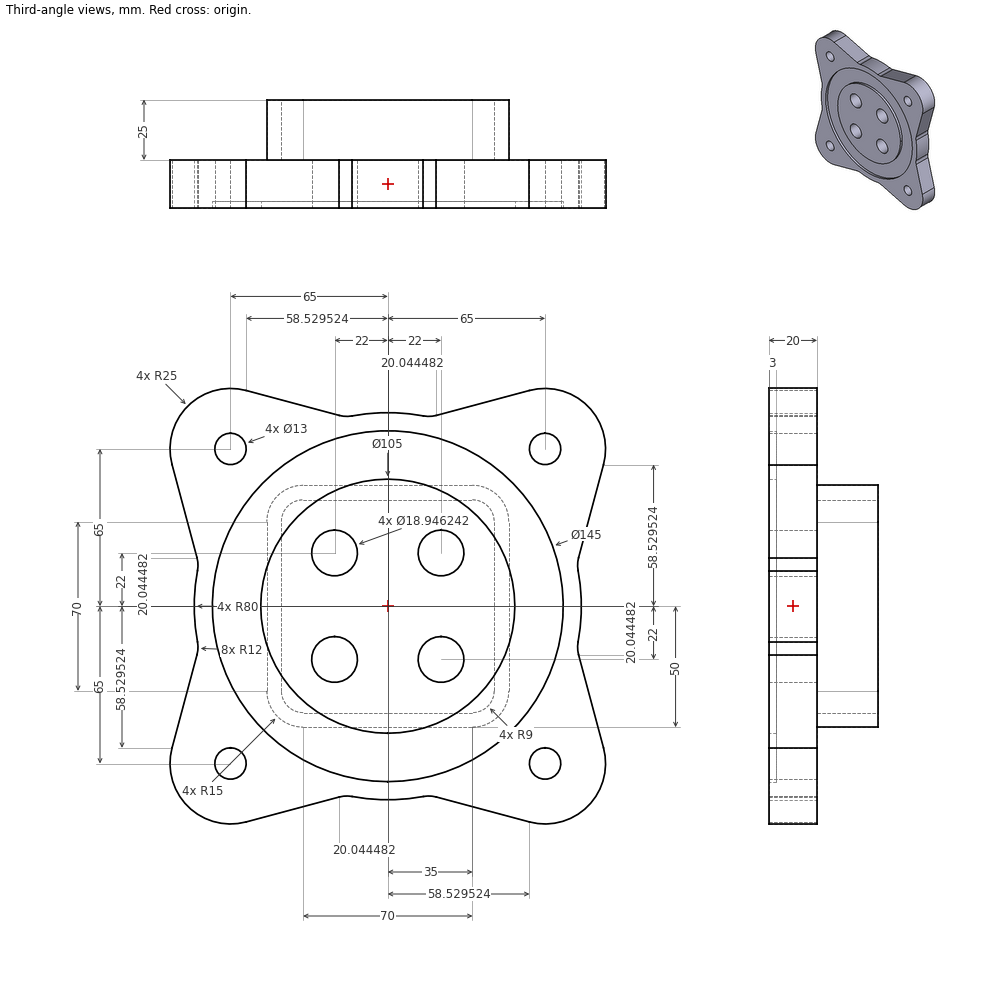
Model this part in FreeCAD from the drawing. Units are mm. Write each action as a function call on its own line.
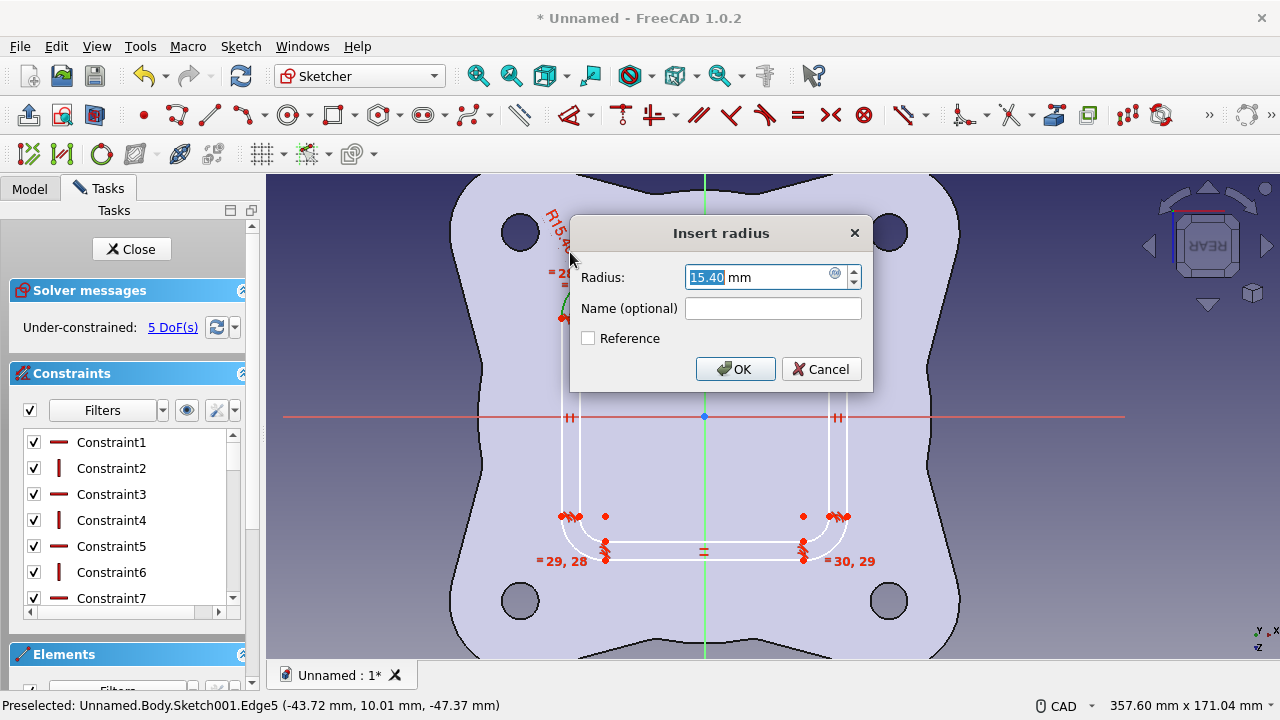
text(15)
key(Return)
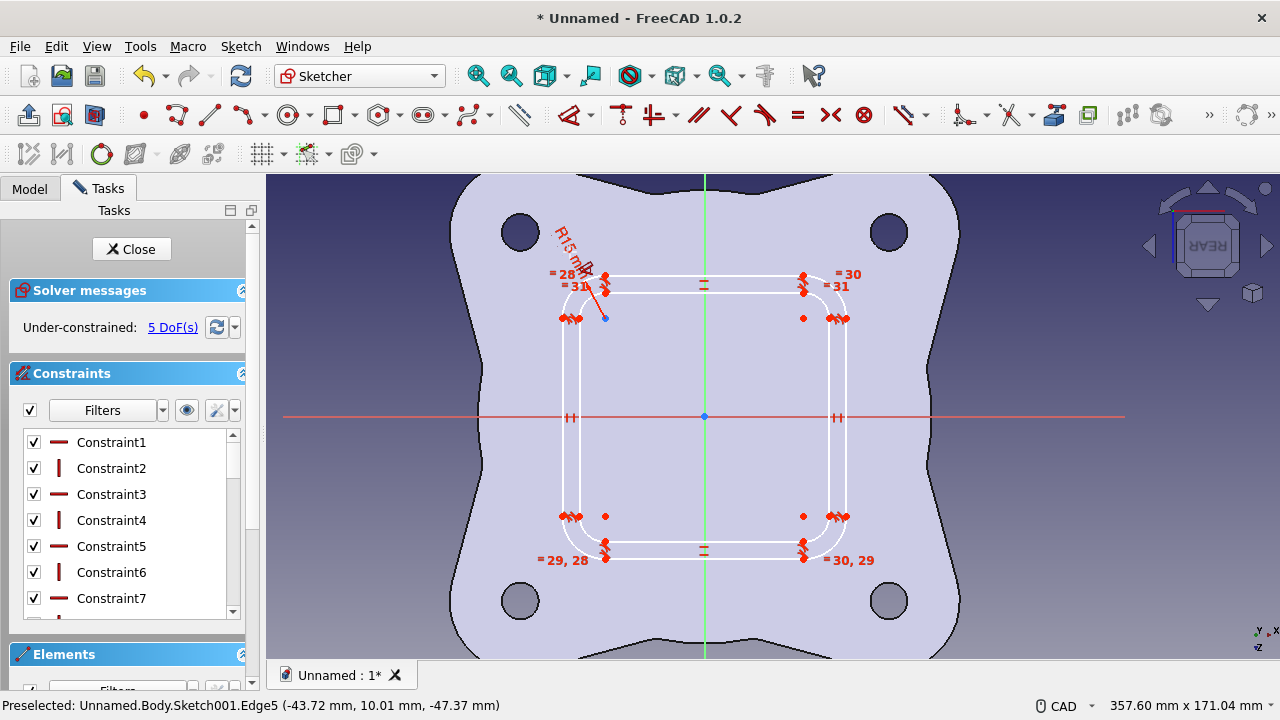
scroll(826, 307, up, 3)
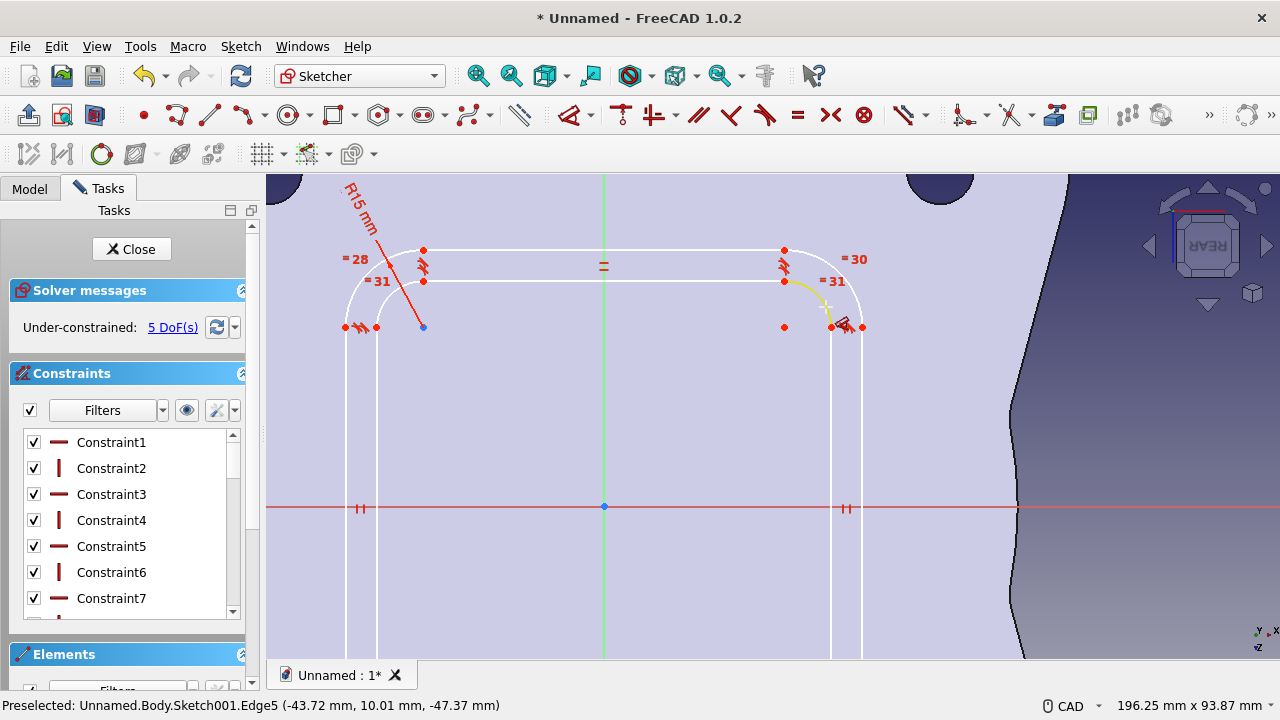
click(826, 307)
click(715, 363)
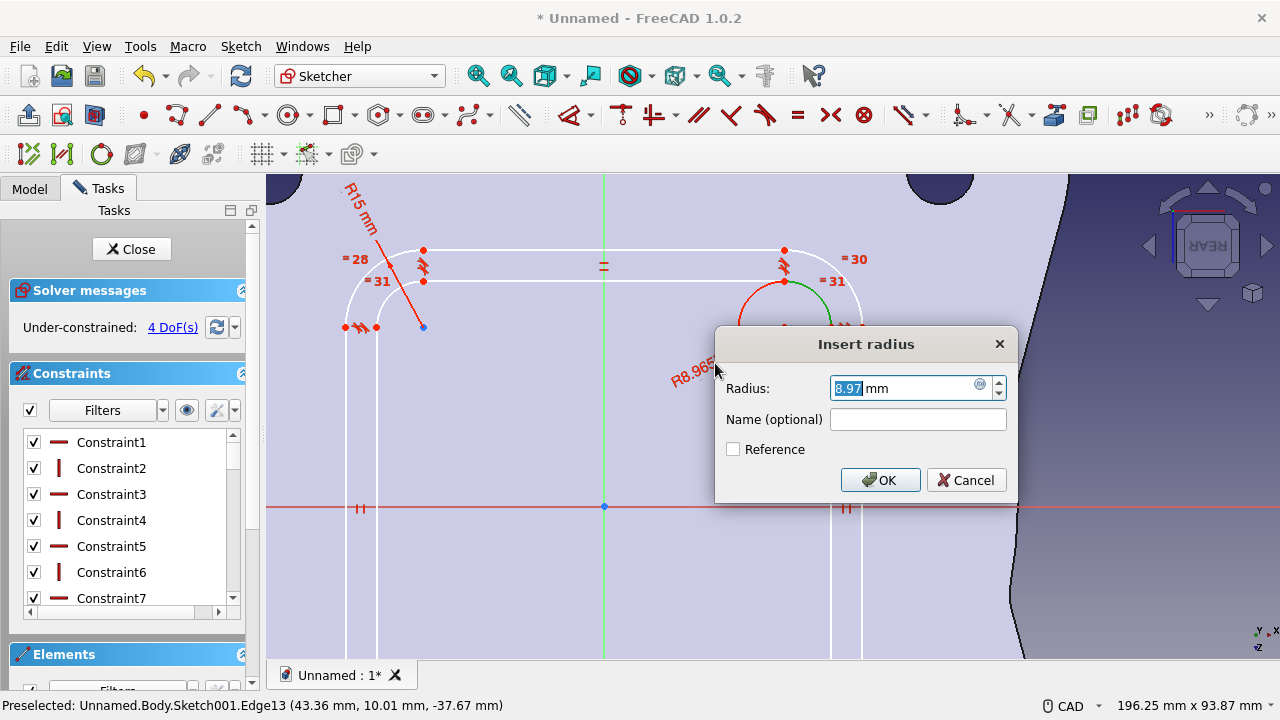
text(9)
key(Return)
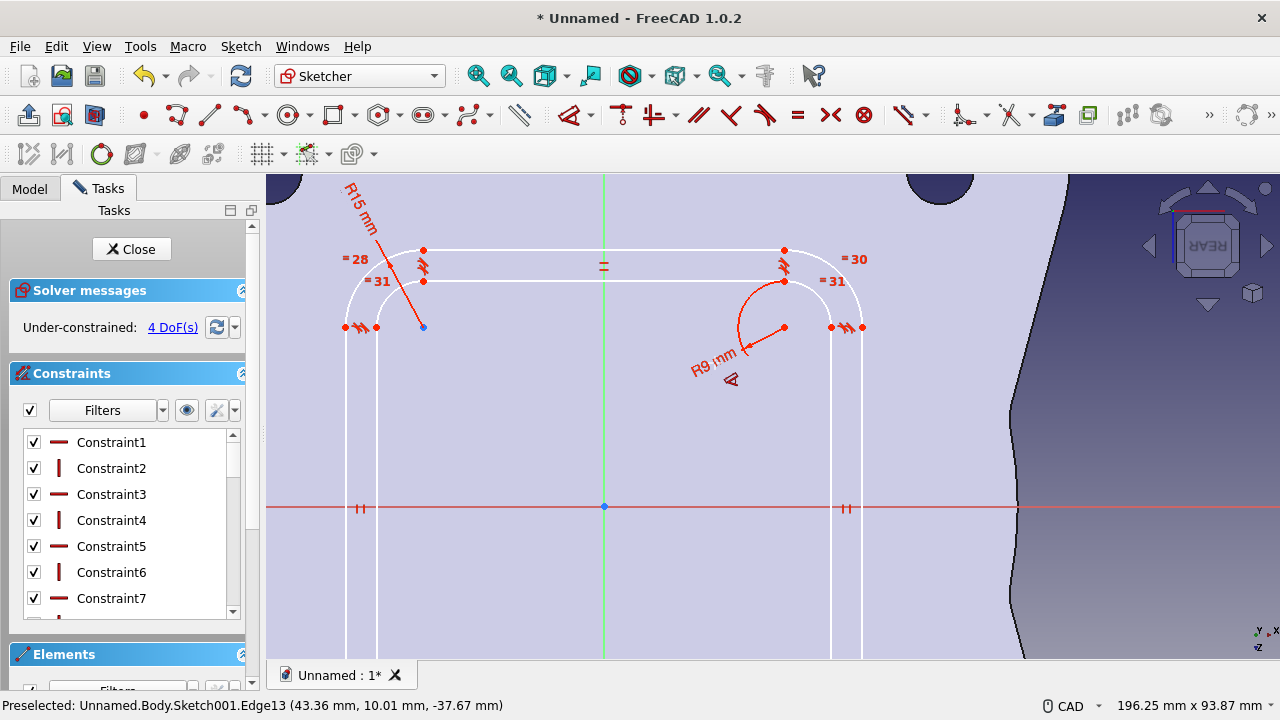
click(676, 250)
click(521, 216)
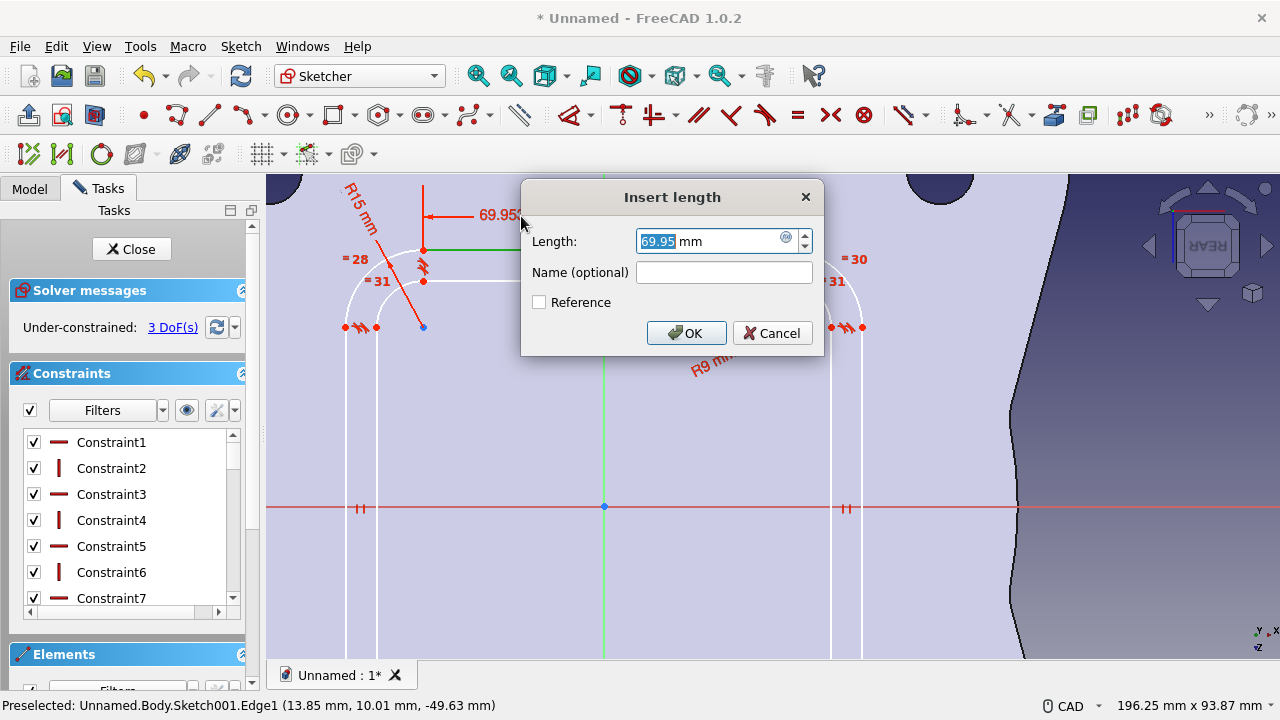
text(70)
key(Return)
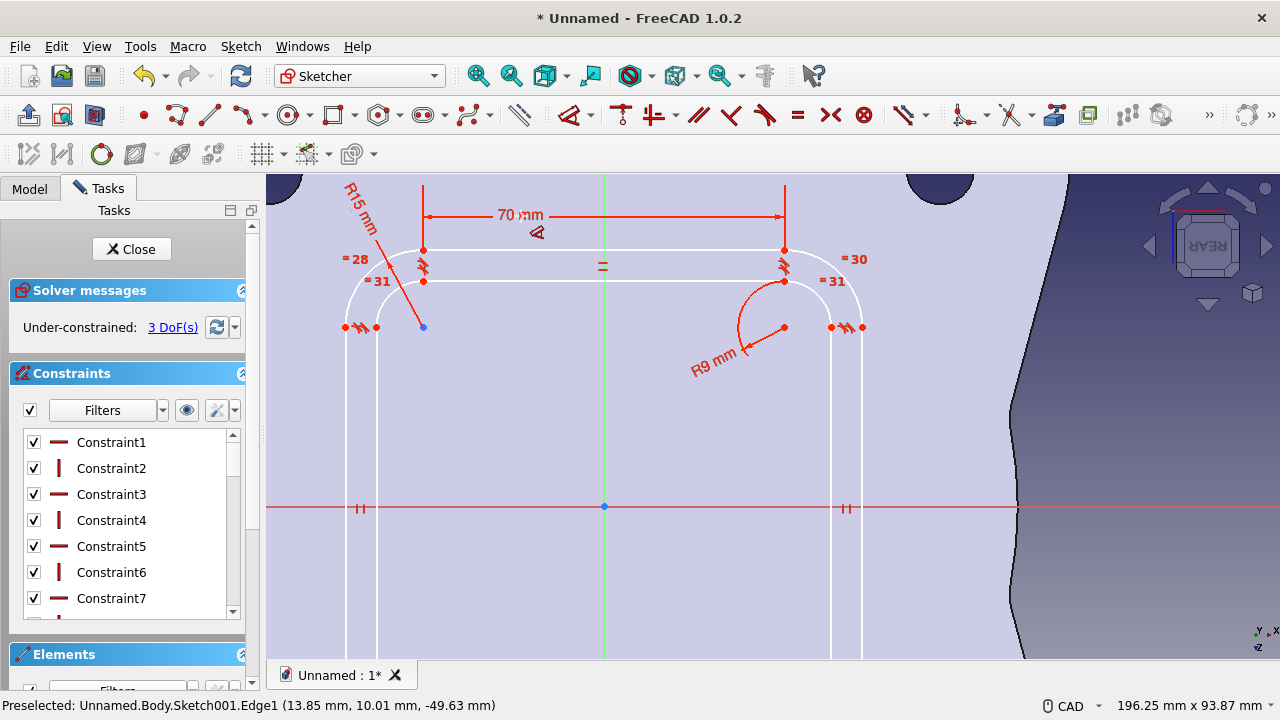
click(346, 436)
click(312, 479)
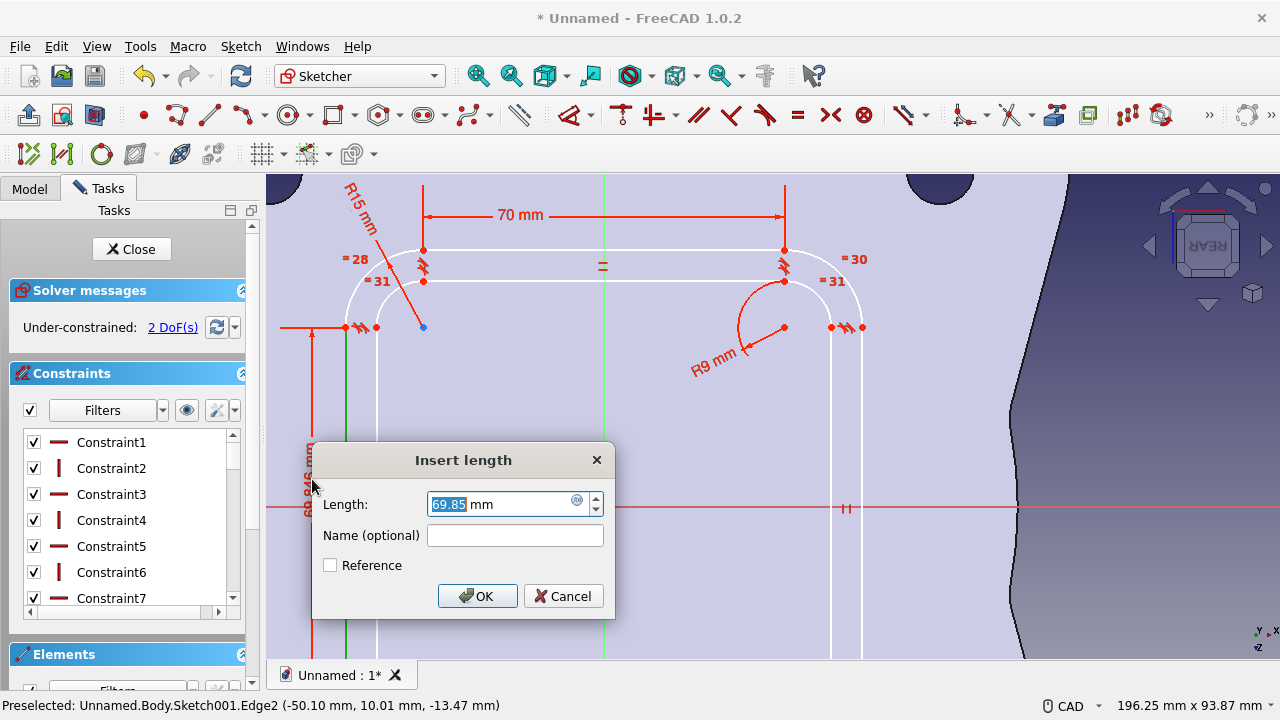
text(70)
key(Return)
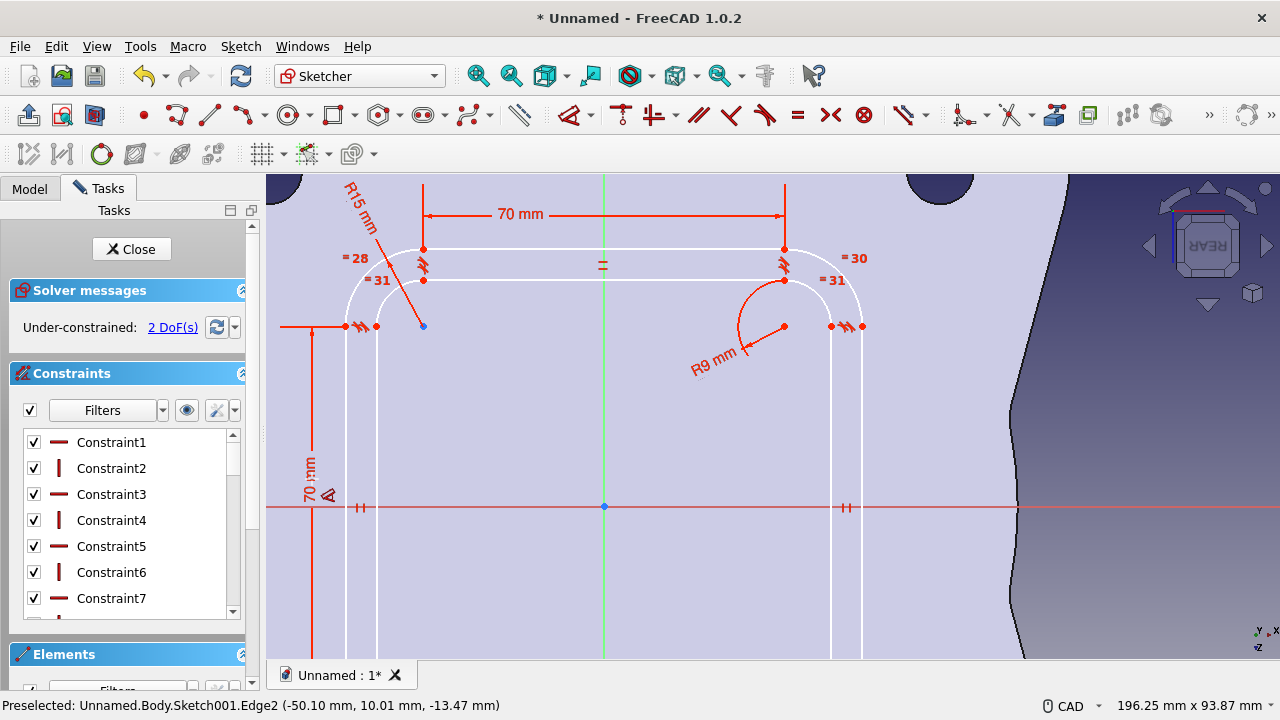
click(785, 249)
click(695, 215)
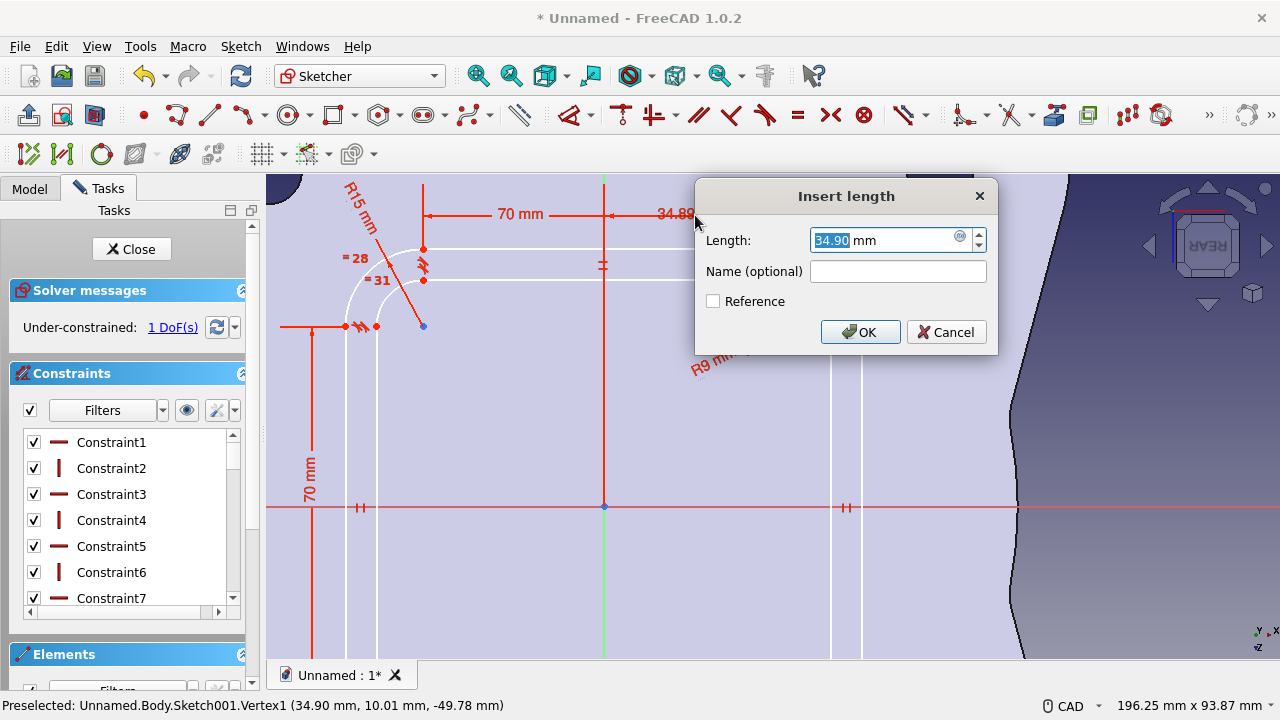
text(35)
key(Return)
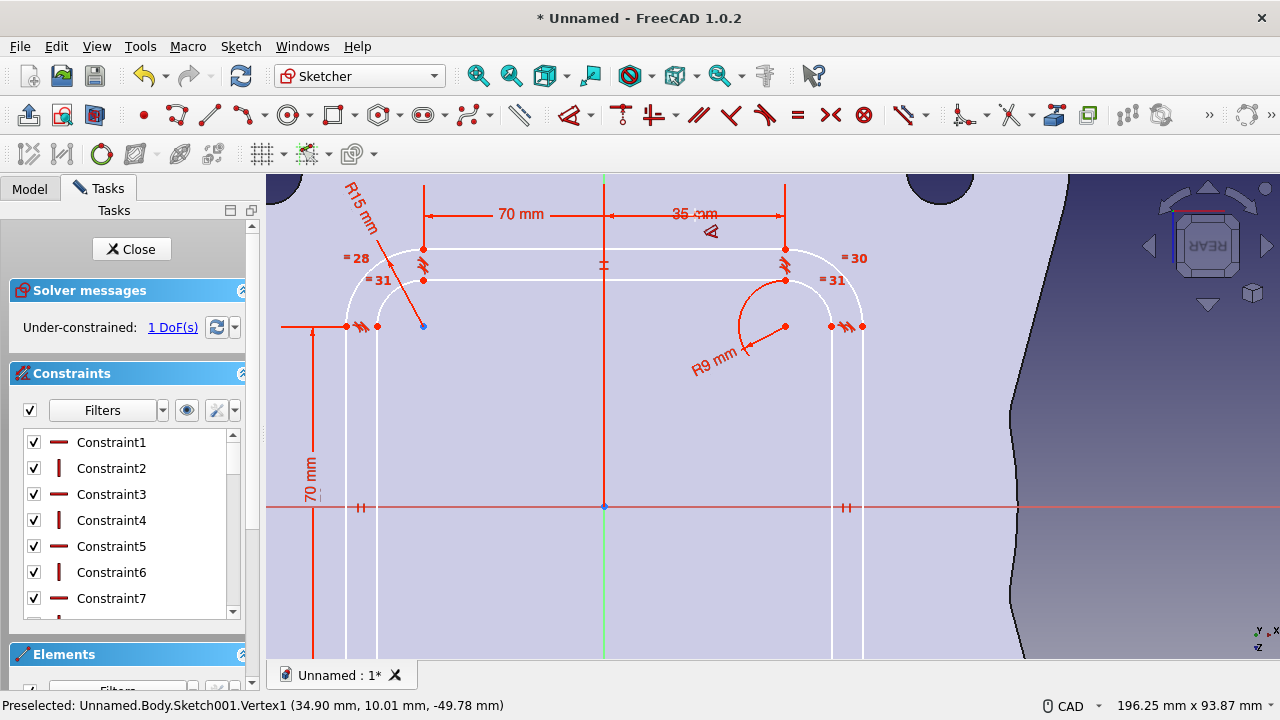
click(785, 249)
click(570, 378)